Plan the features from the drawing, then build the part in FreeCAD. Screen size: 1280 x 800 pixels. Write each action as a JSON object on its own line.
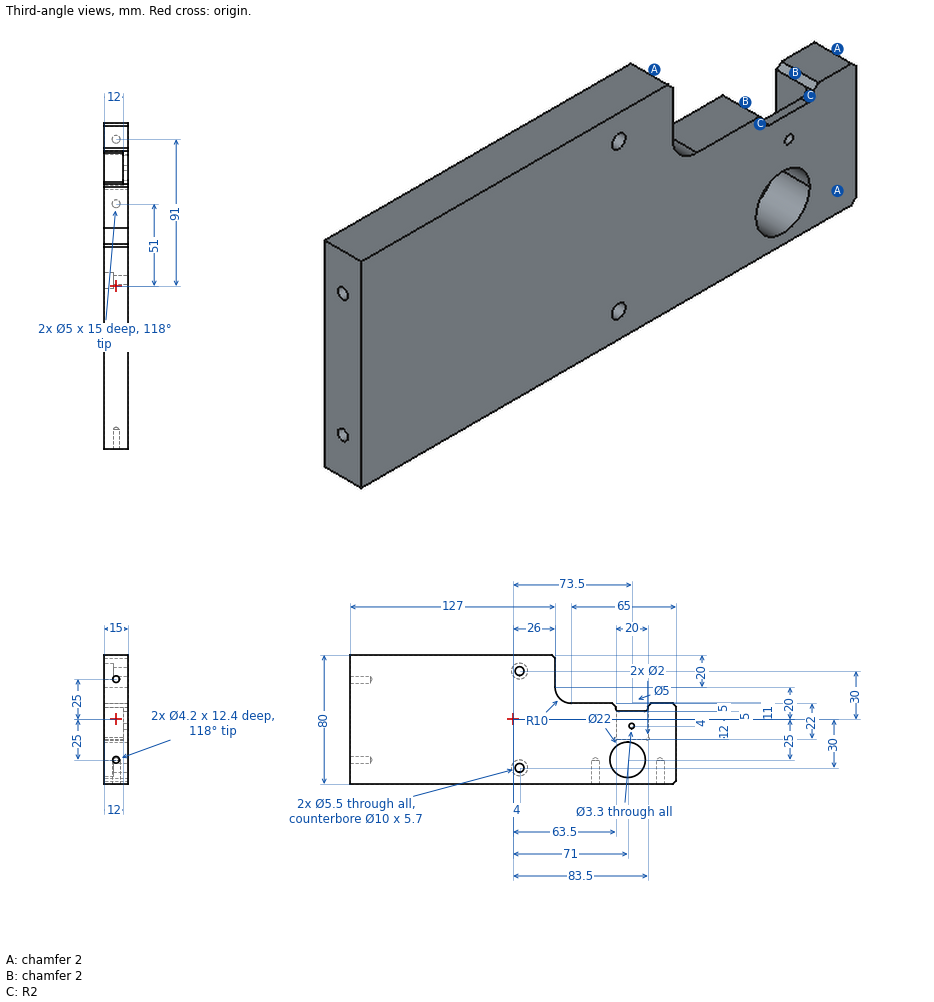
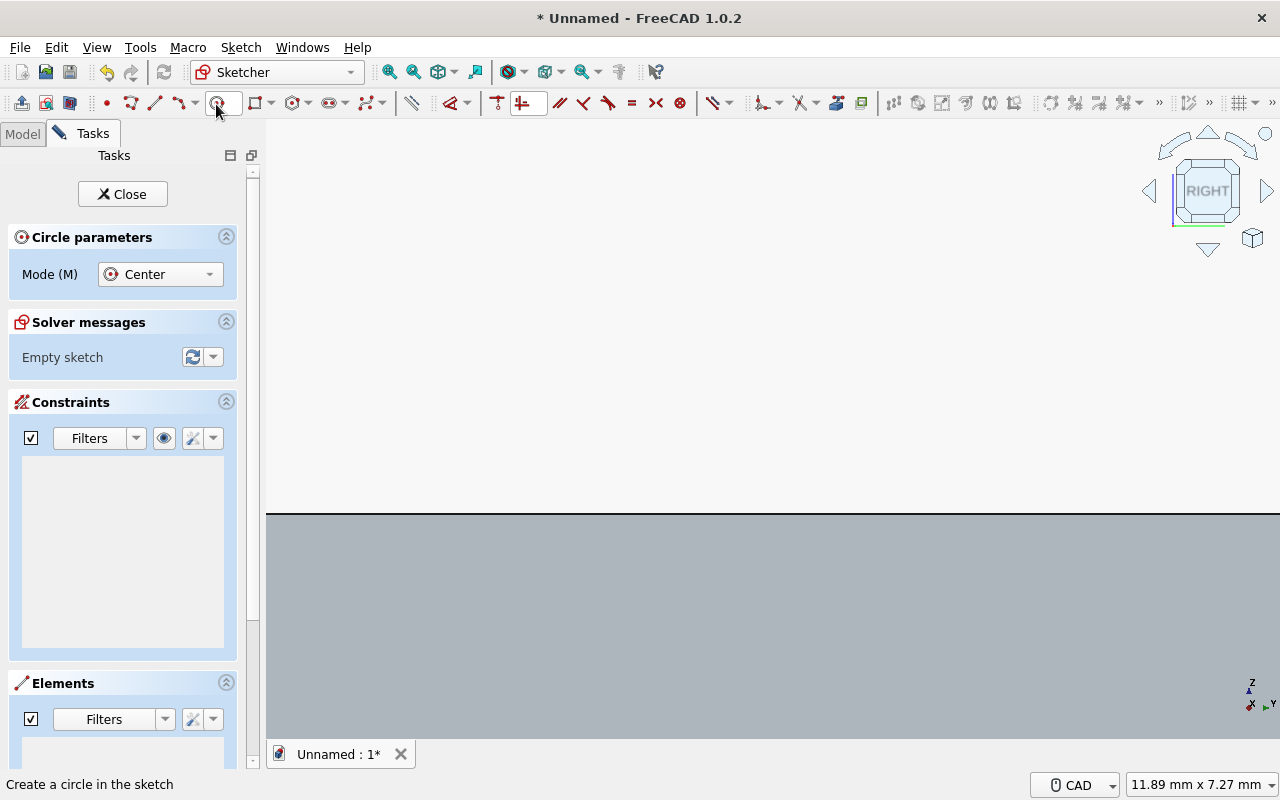
{"action": "left_click", "coordinate": [704, 429]}
{"action": "left_click", "coordinate": [855, 278]}
{"action": "key", "text": "Escape"}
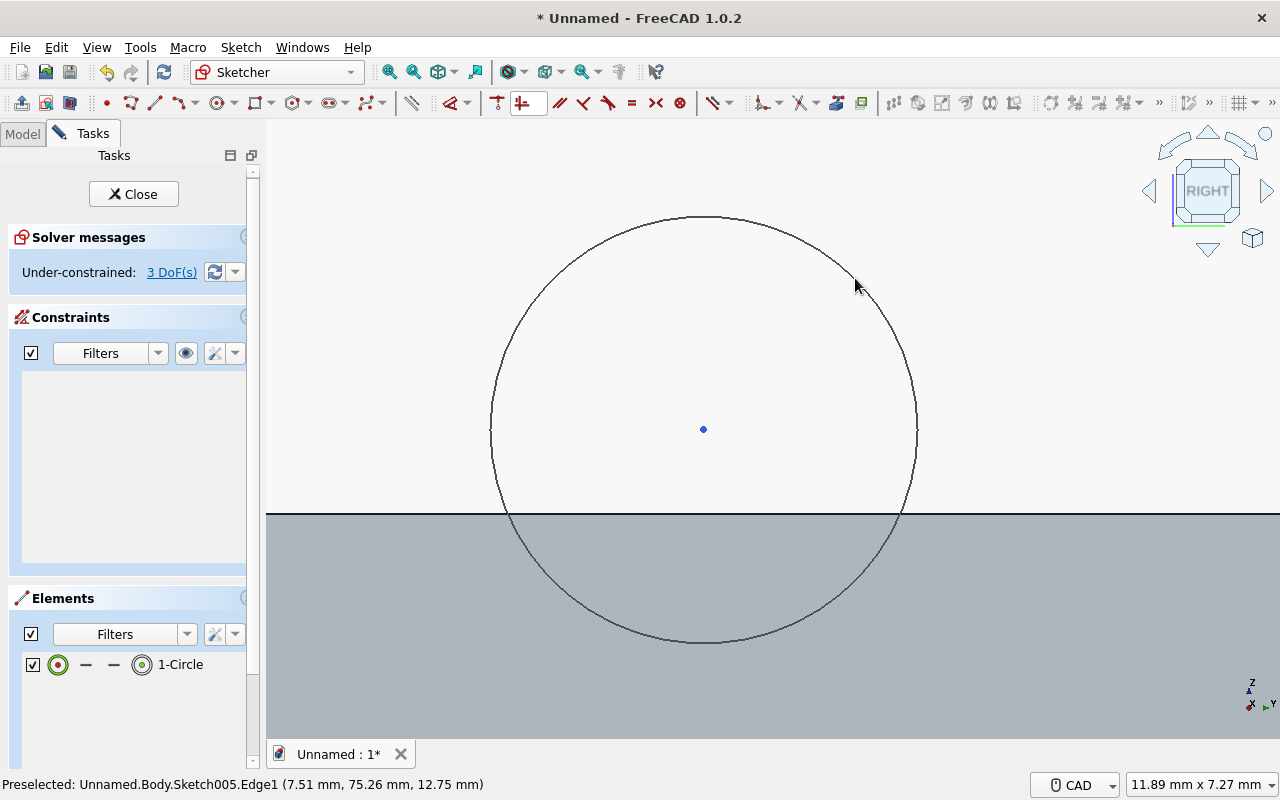
{"action": "left_click", "coordinate": [450, 104]}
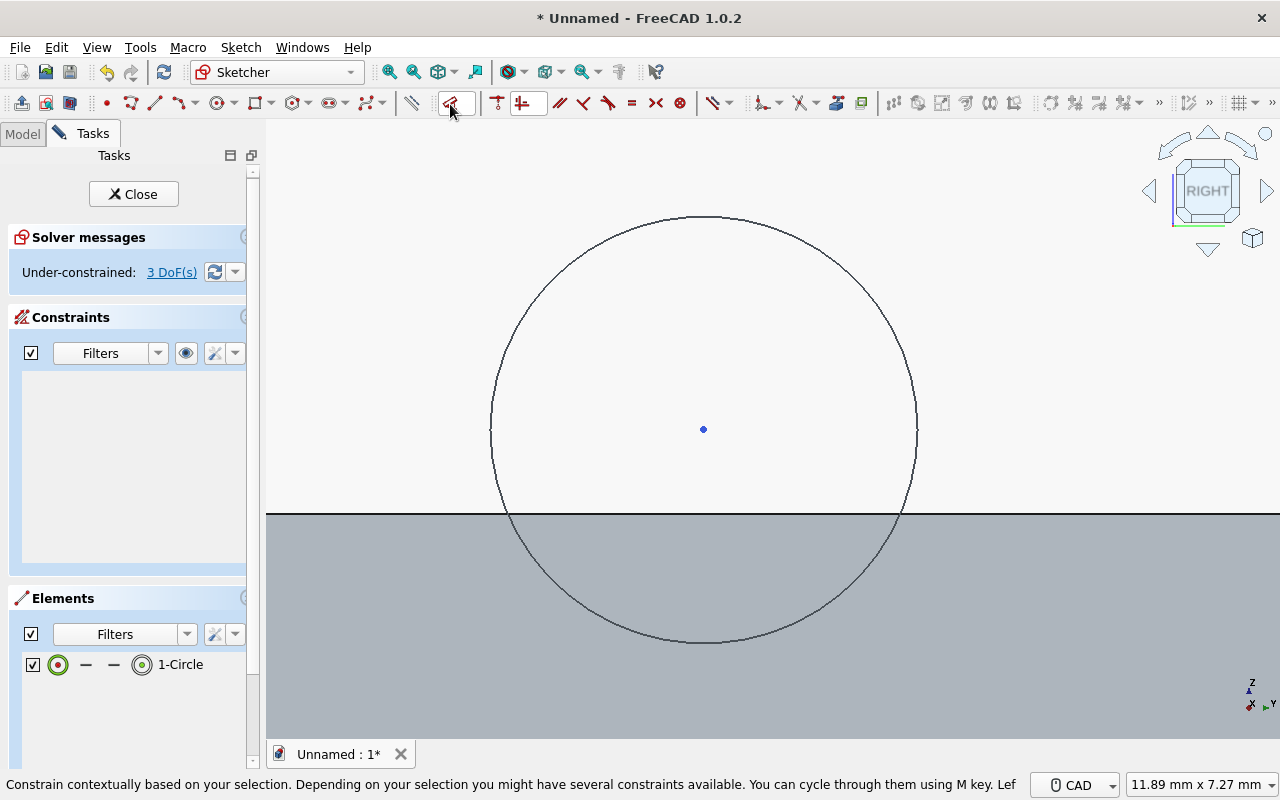
{"action": "left_click", "coordinate": [855, 279]}
{"action": "left_click", "coordinate": [878, 256]}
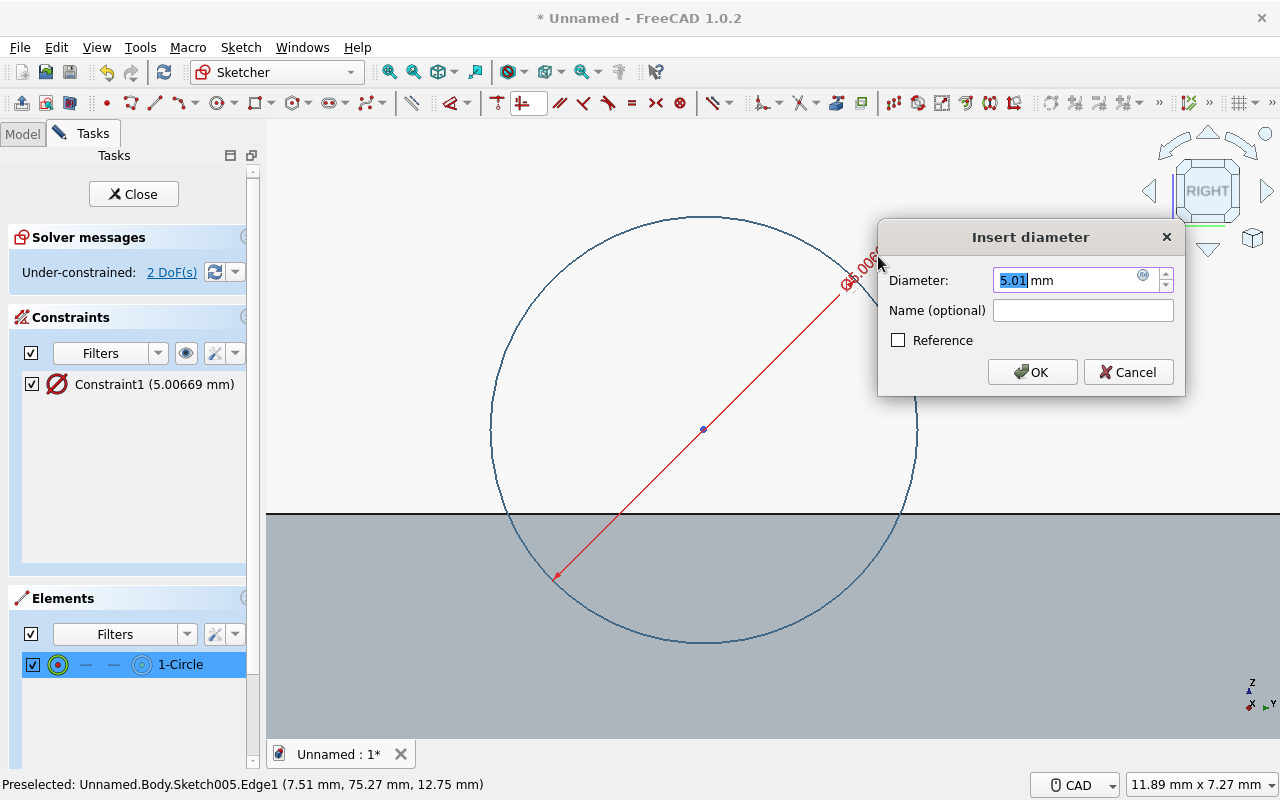
{"action": "type", "text": "5"}
{"action": "key", "text": "Return"}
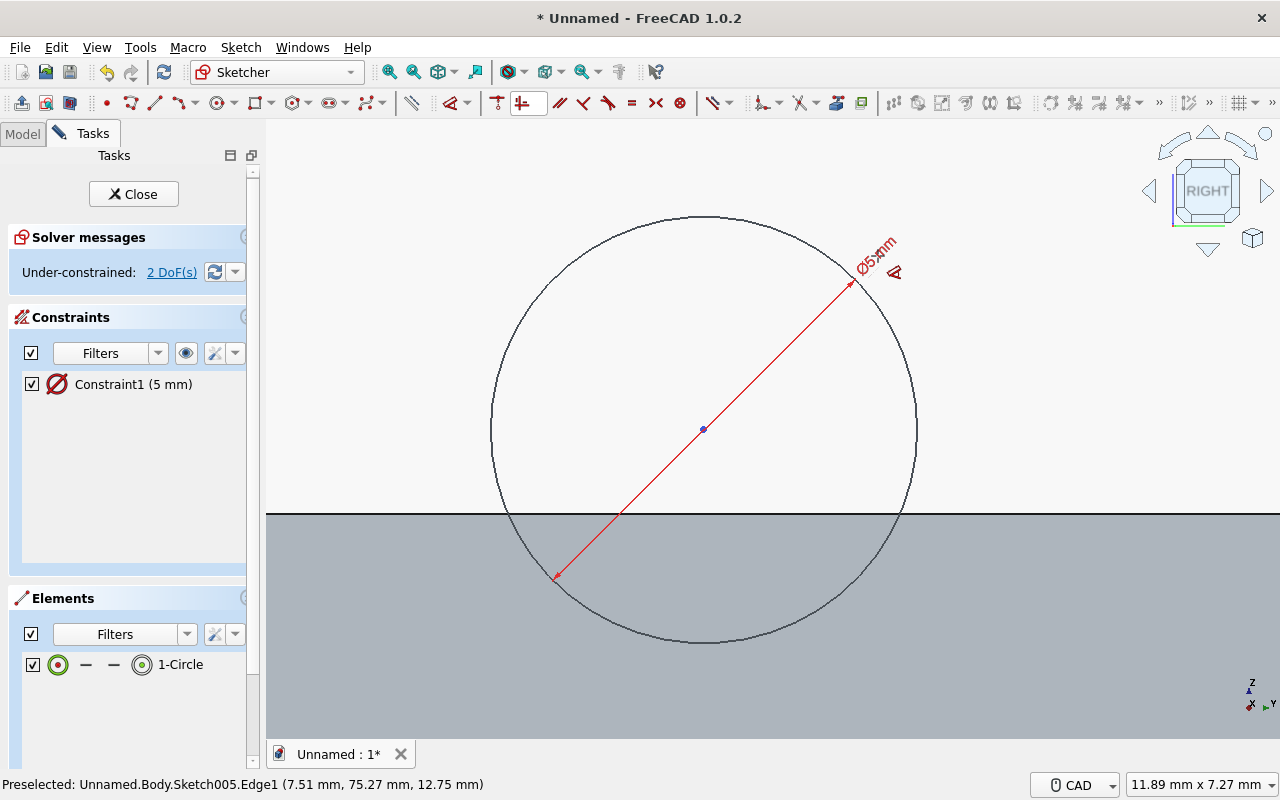
{"action": "left_click", "coordinate": [704, 430]}
{"action": "left_click", "coordinate": [738, 571]}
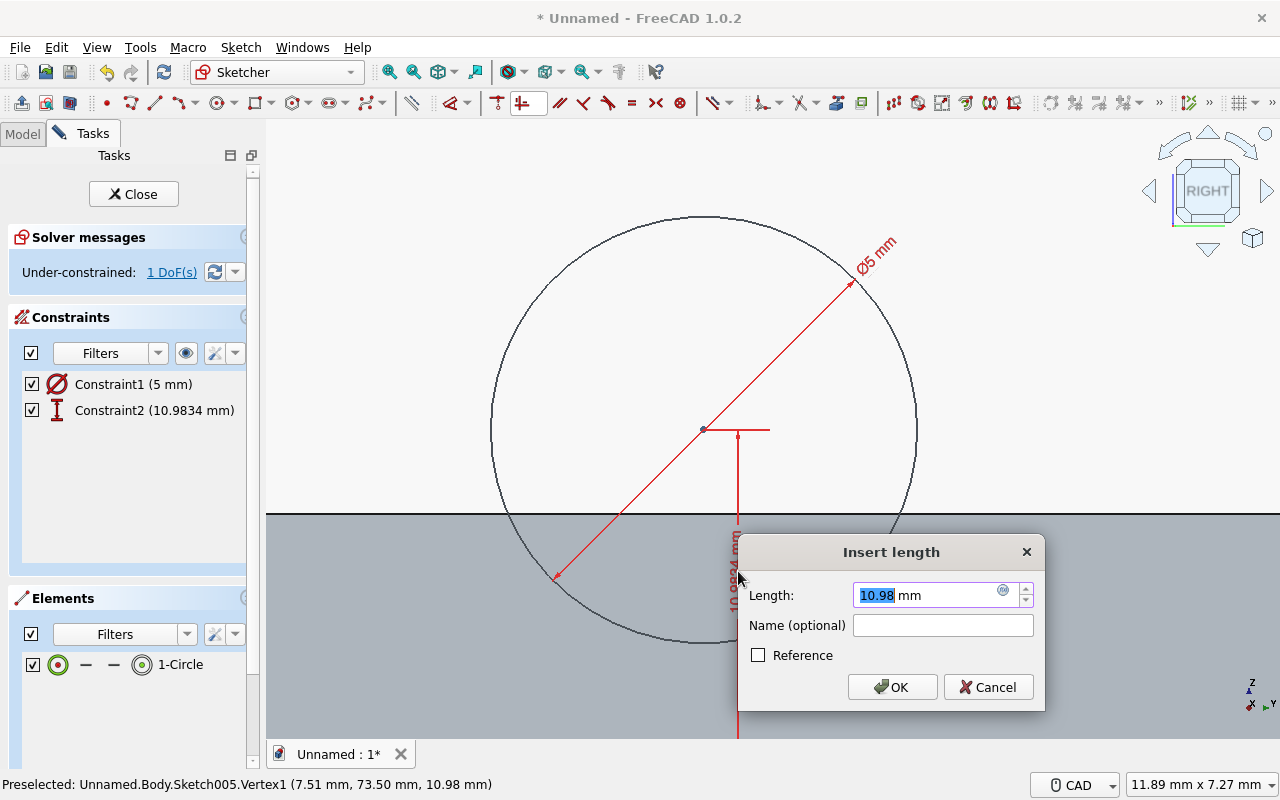
{"action": "type", "text": "11"}
{"action": "key", "text": "Return"}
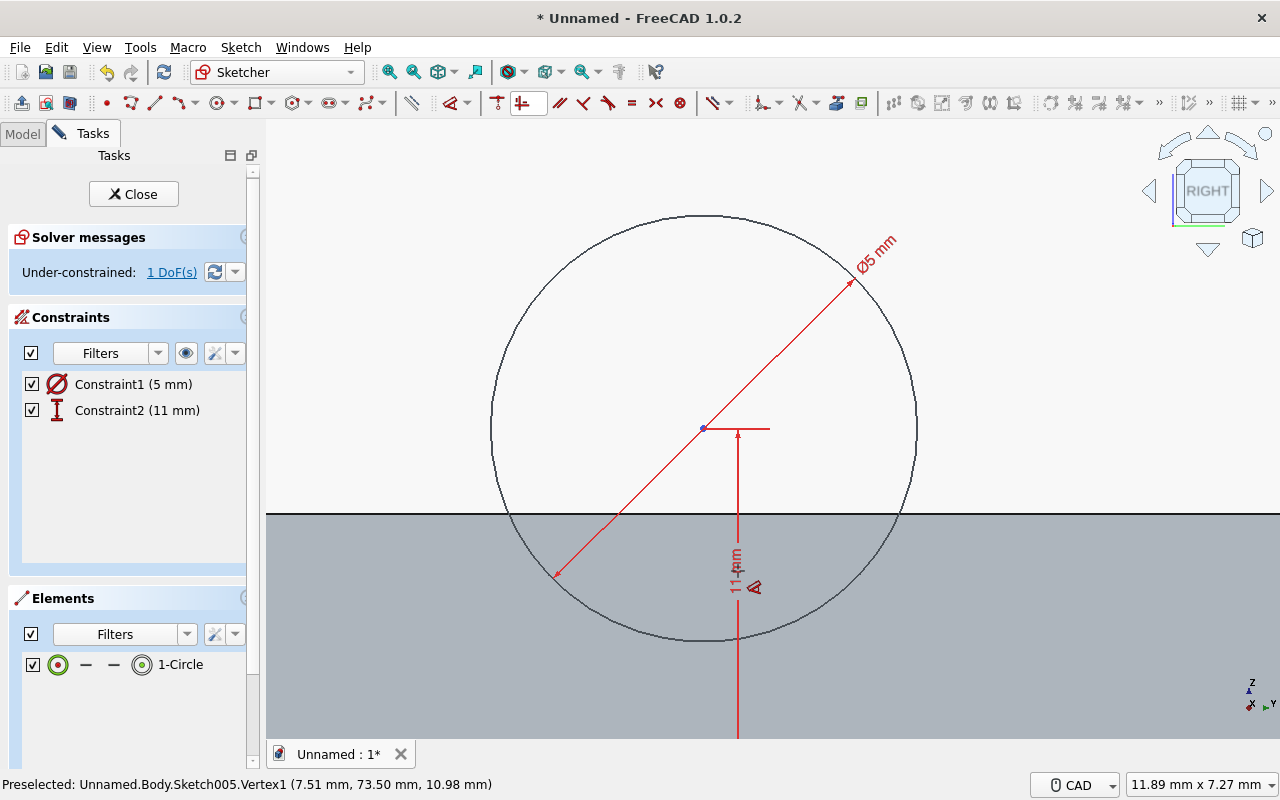
{"action": "left_click", "coordinate": [704, 429]}
{"action": "left_click", "coordinate": [405, 395]}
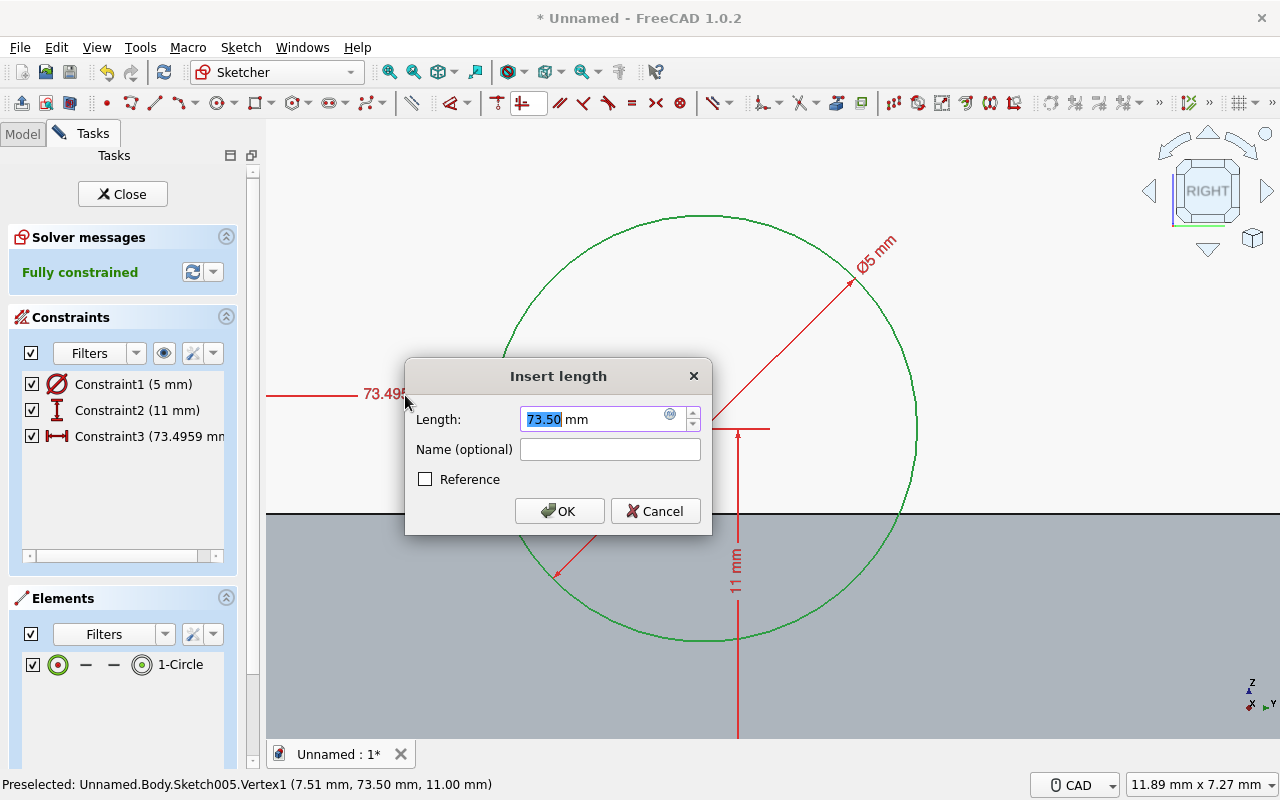
{"action": "type", "text": "73.5"}
{"action": "key", "text": "Return"}
{"action": "key", "text": "Escape"}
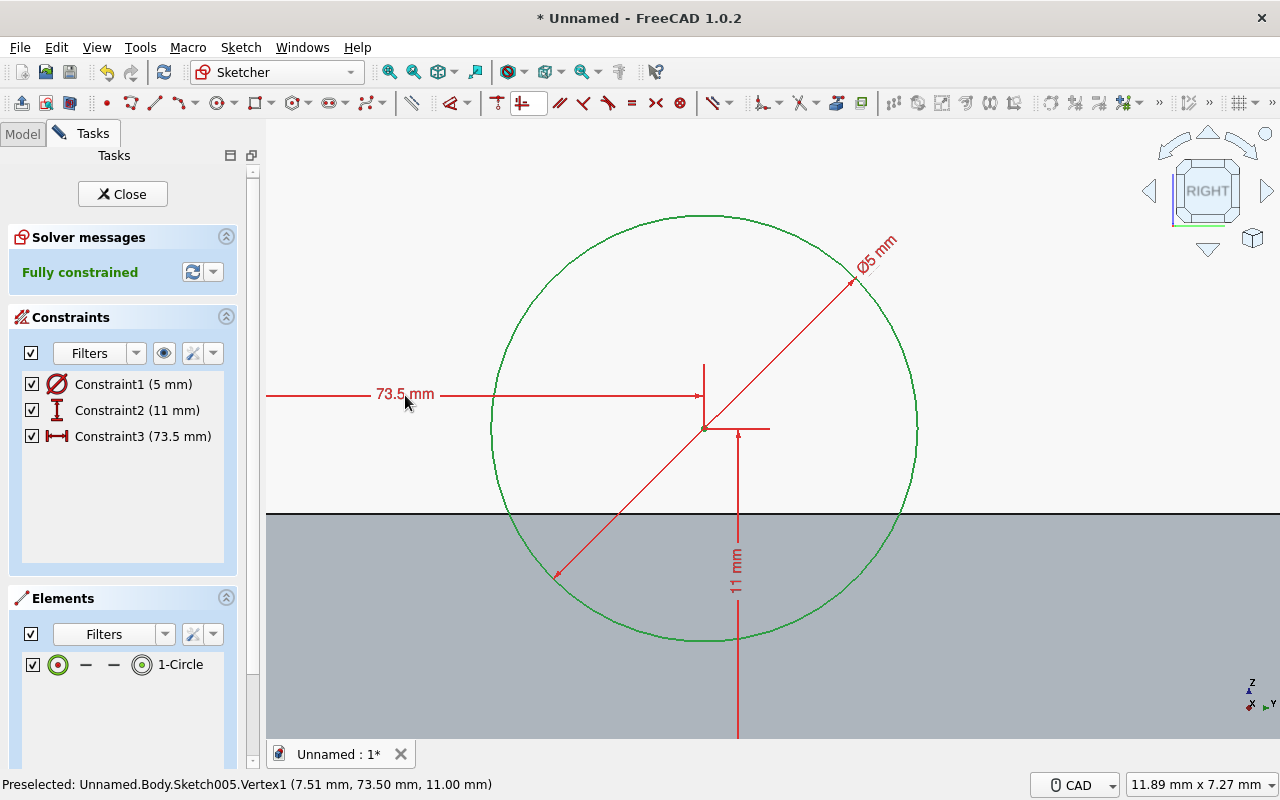
{"action": "left_click", "coordinate": [123, 194]}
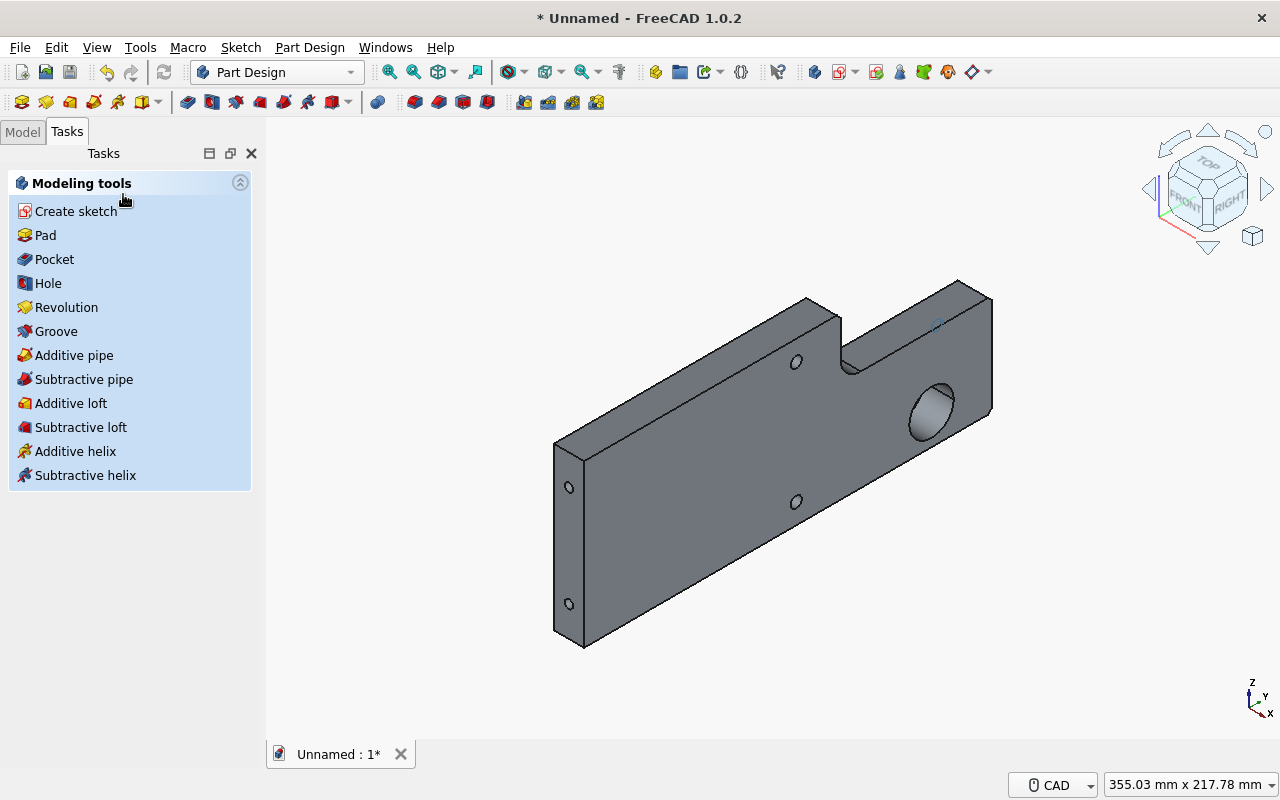
{"action": "left_click", "coordinate": [188, 102]}